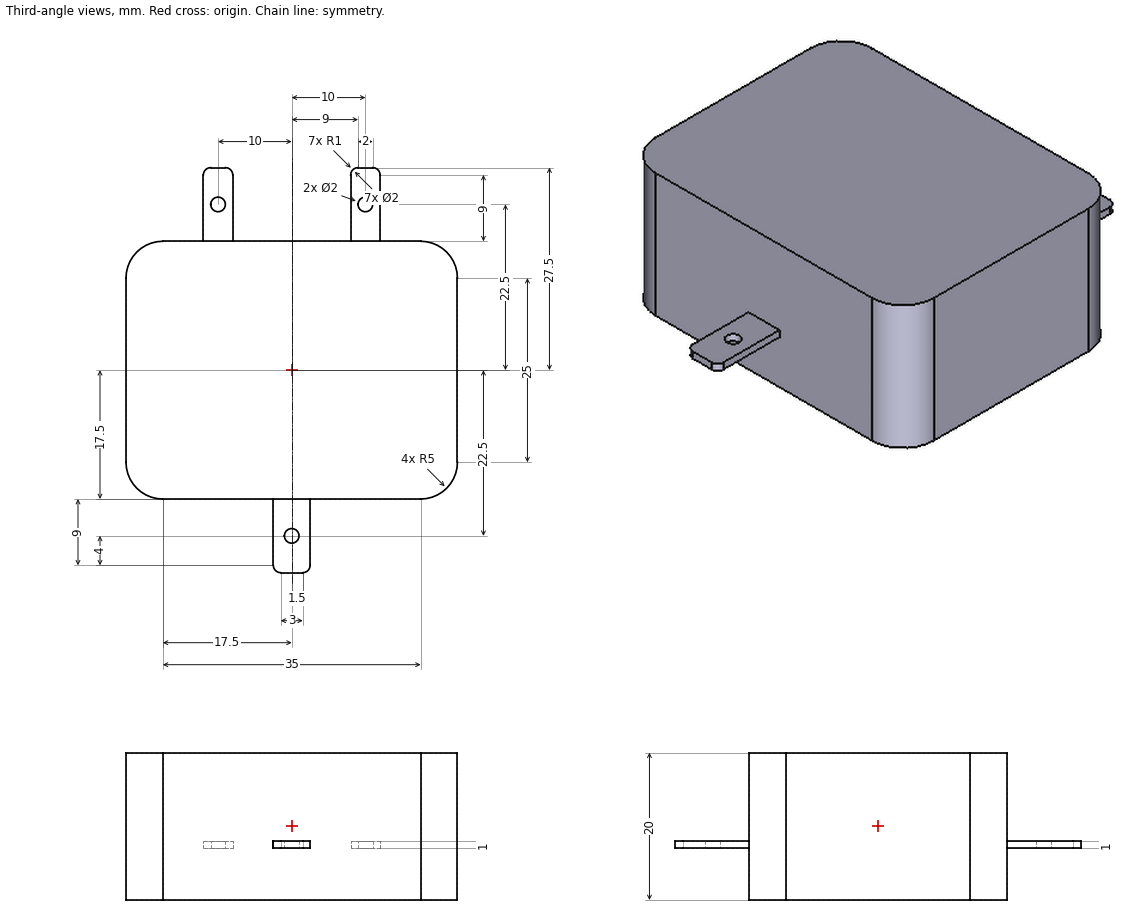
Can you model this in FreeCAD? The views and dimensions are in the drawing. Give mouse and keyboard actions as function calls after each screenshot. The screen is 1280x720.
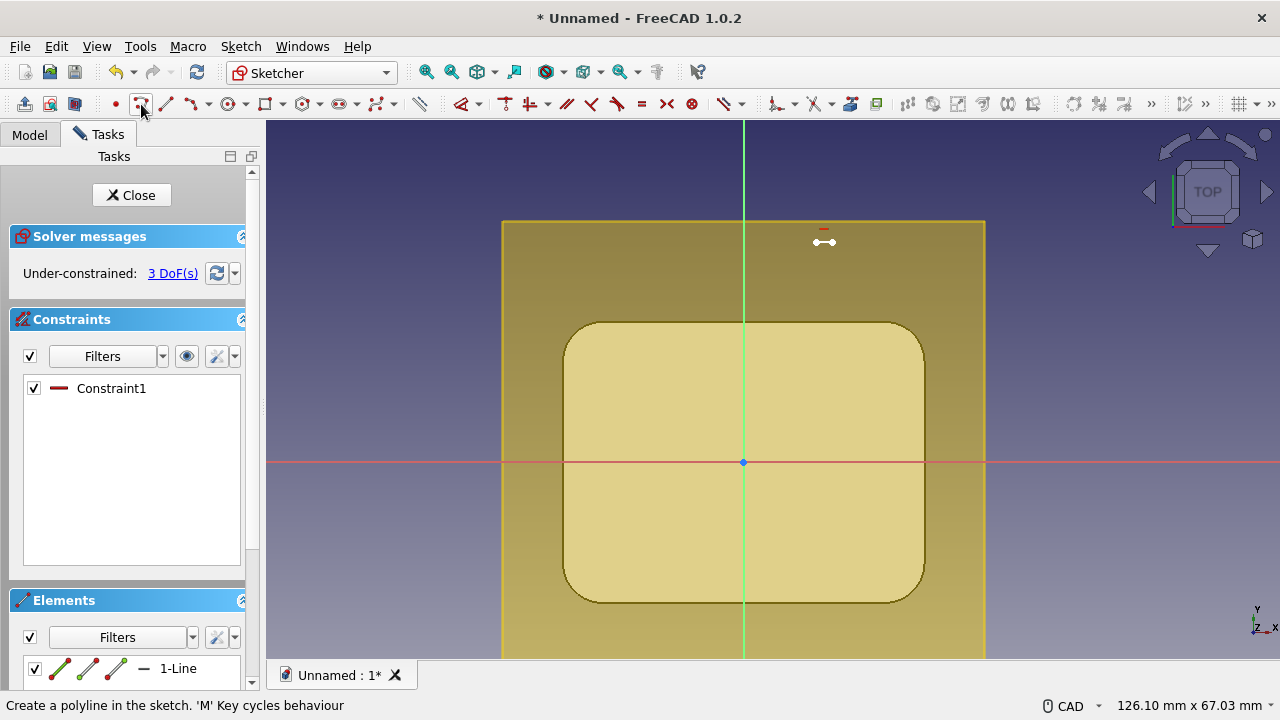
scroll(840, 249, up, 2)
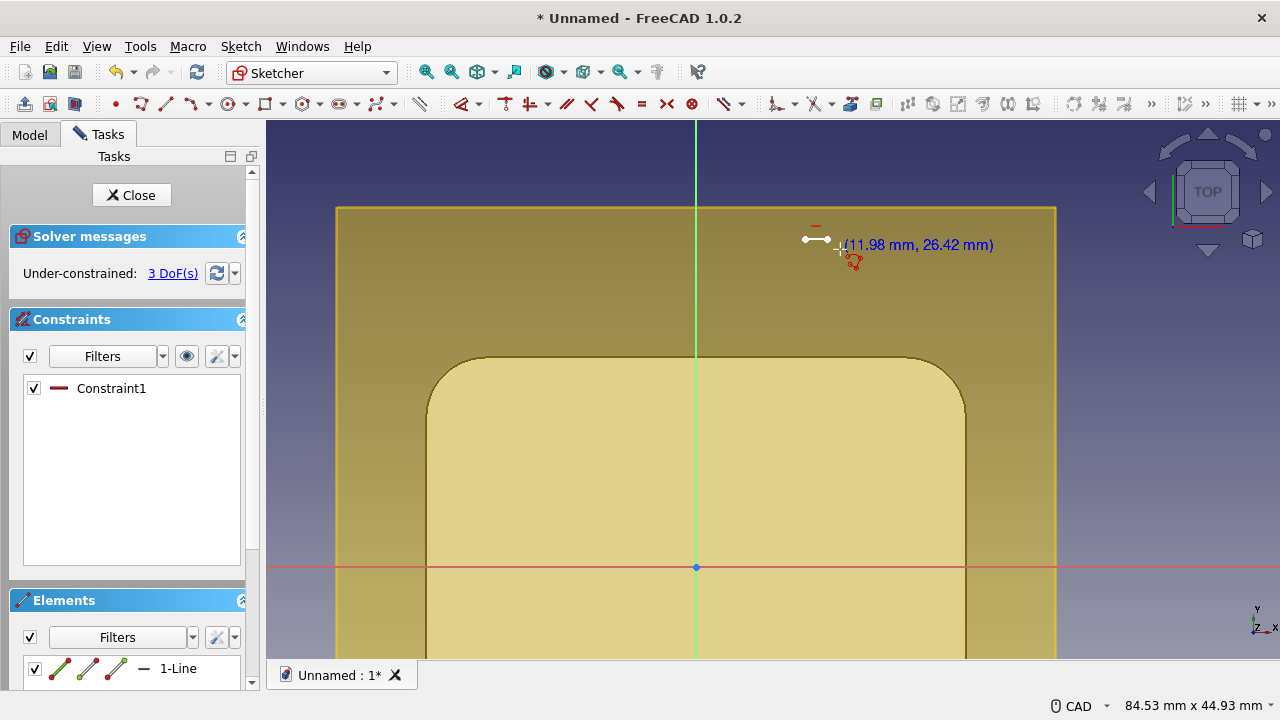
click(840, 249)
click(840, 357)
click(792, 357)
click(792, 249)
right_click(792, 249)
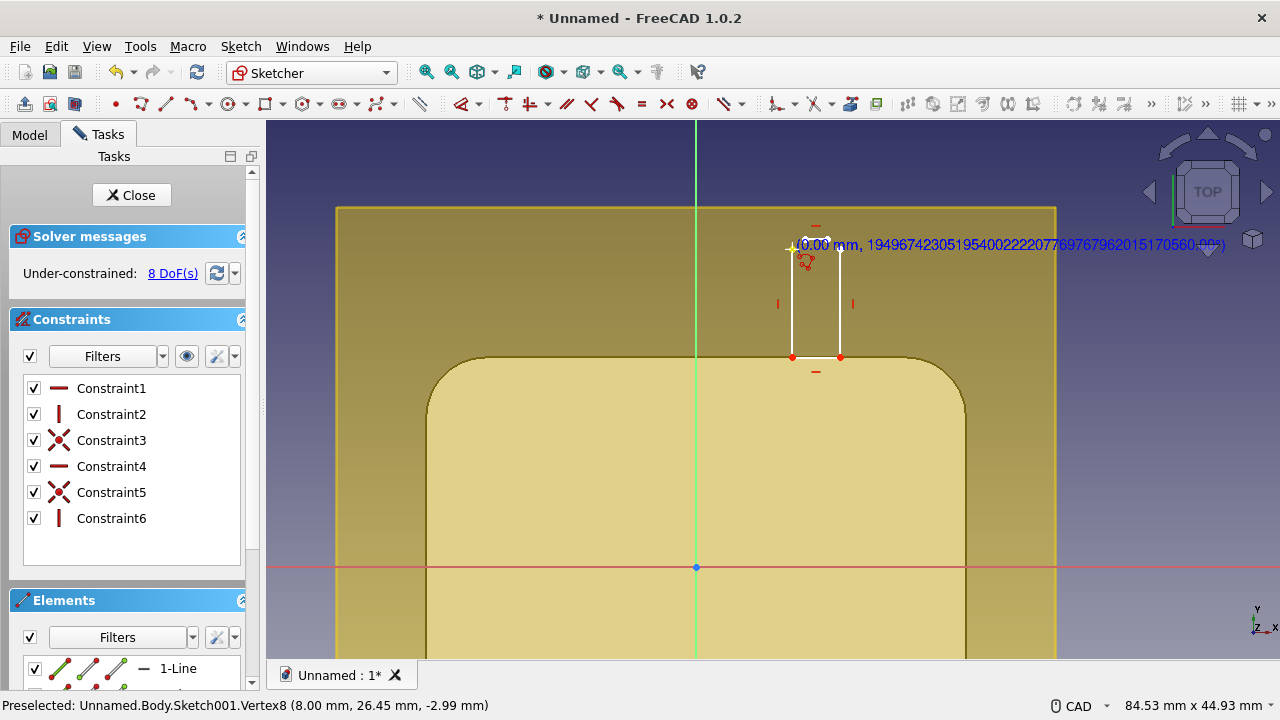
click(190, 104)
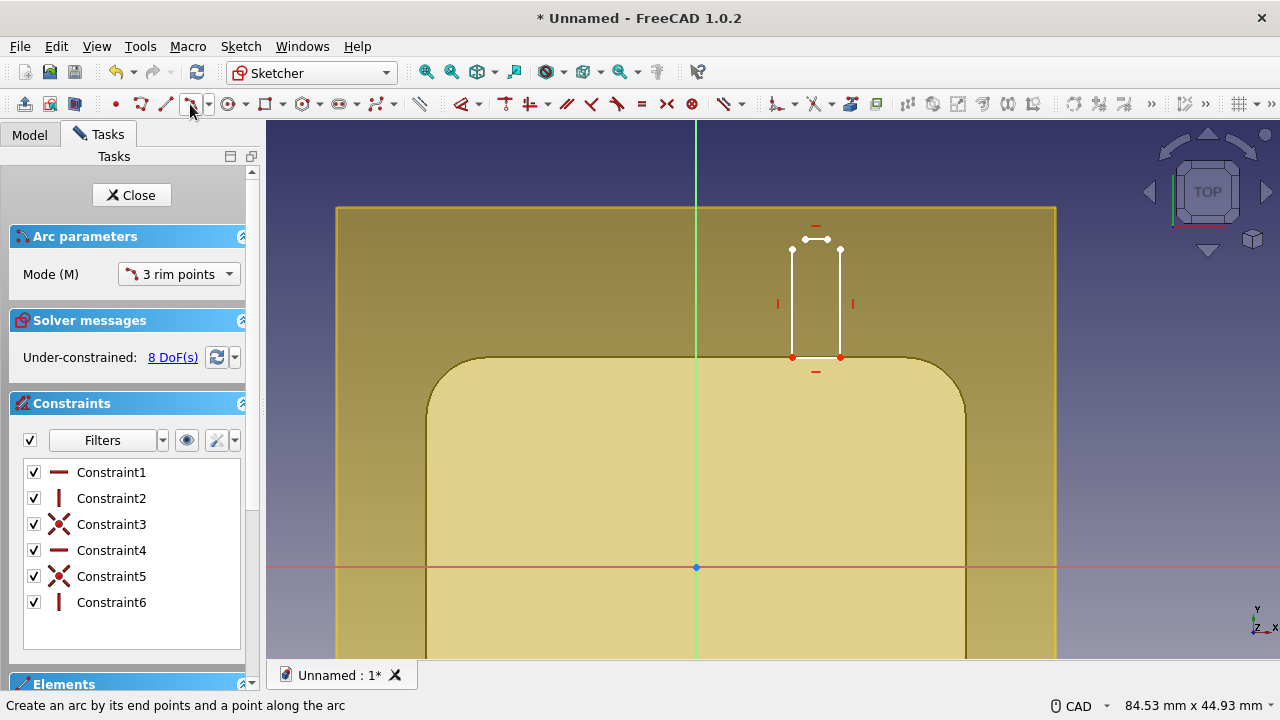
scroll(828, 237, up, 2)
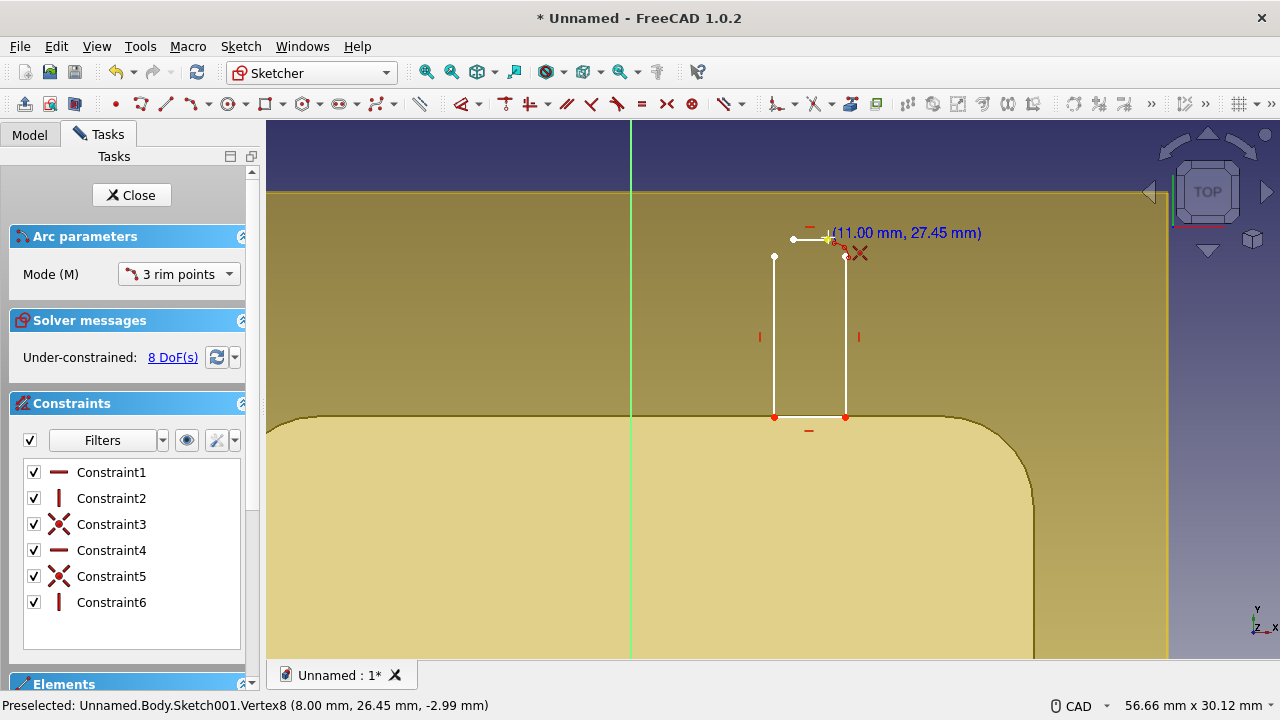
click(827, 240)
click(846, 256)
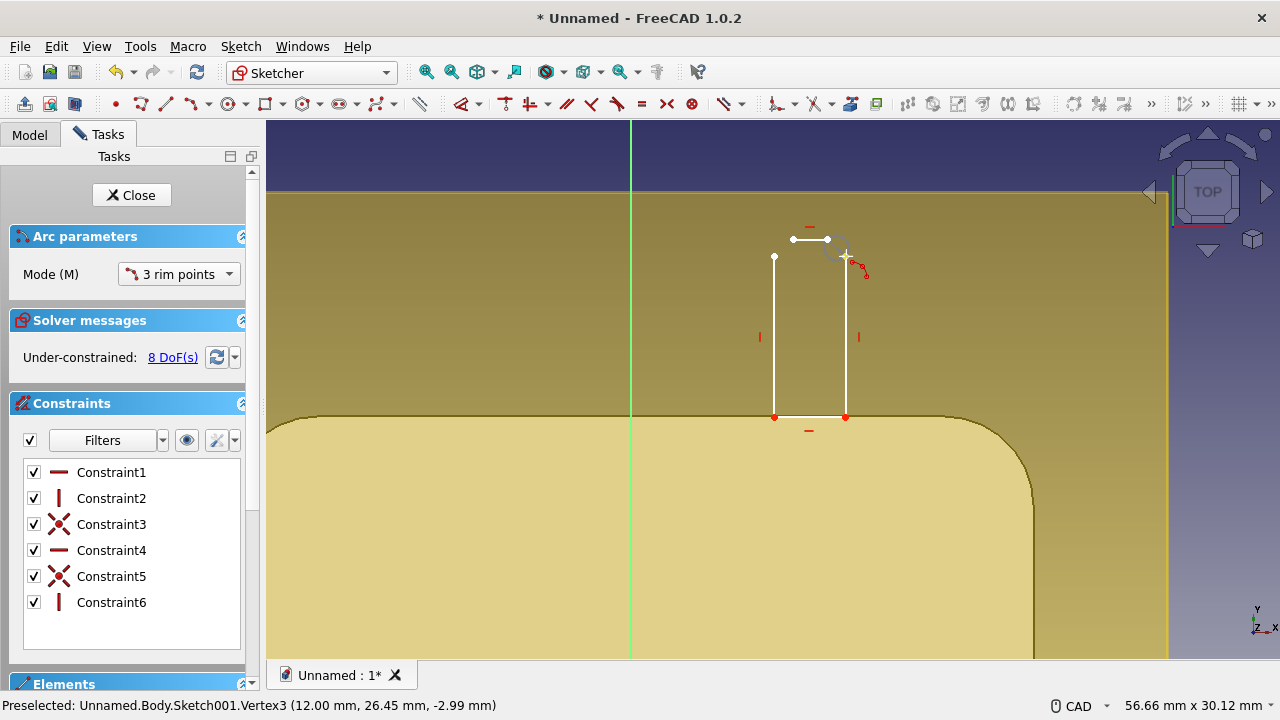
scroll(840, 243, up, 6)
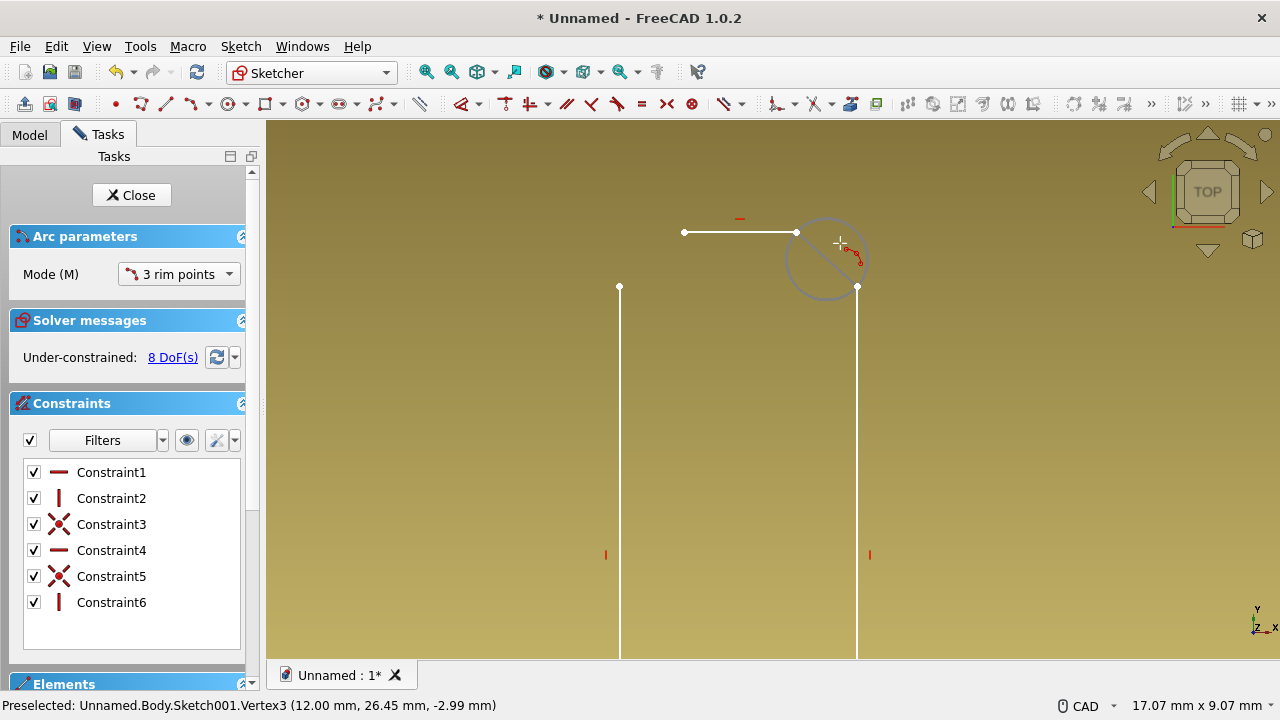
click(840, 242)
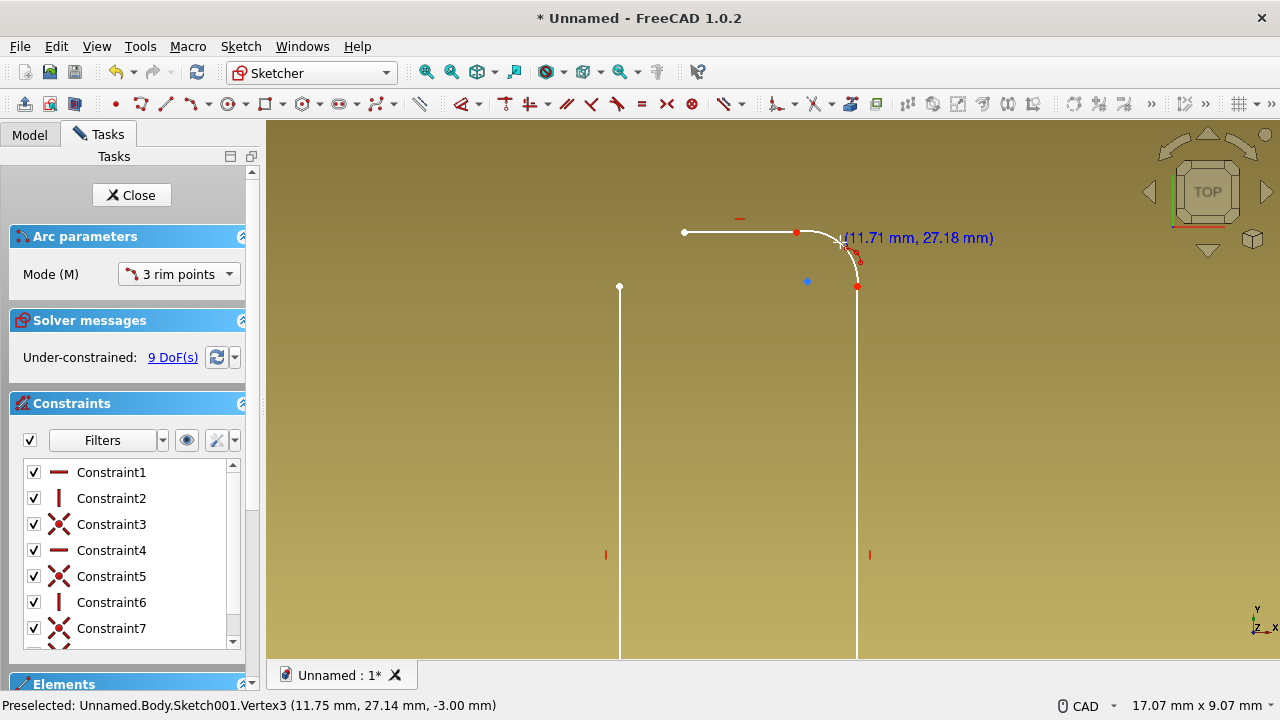
scroll(774, 207, down, 11)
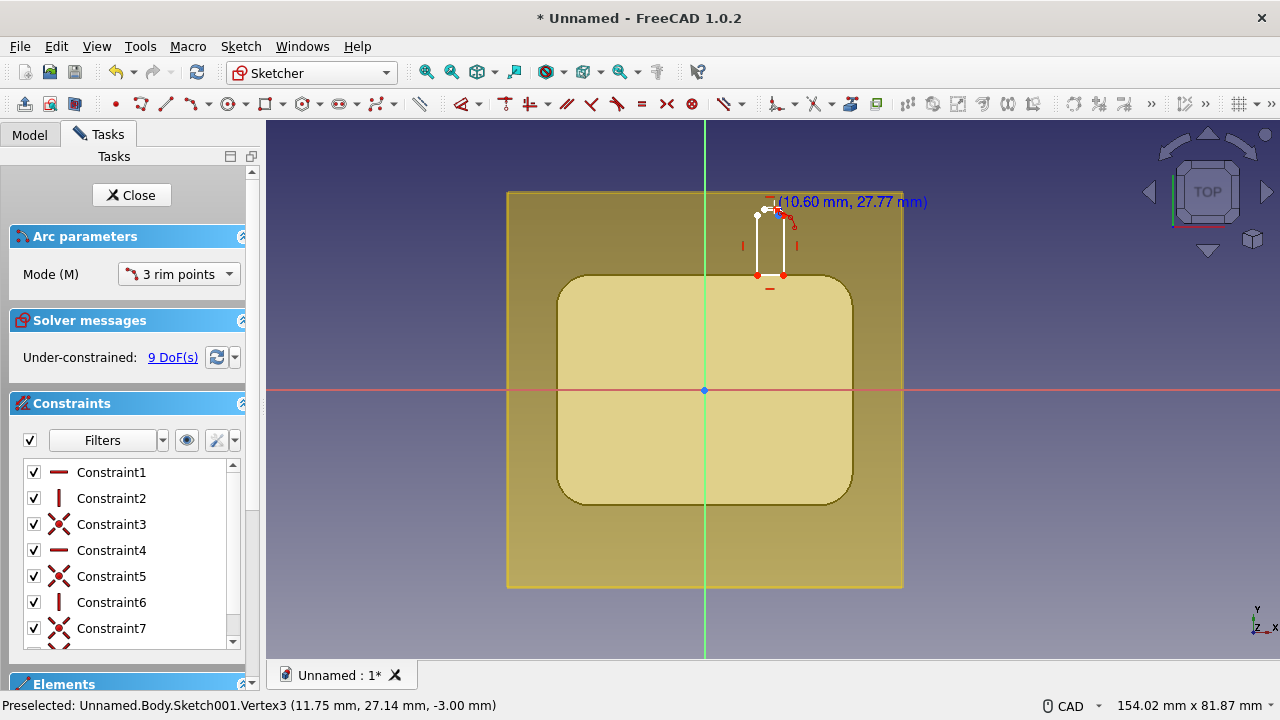
scroll(757, 216, up, 3)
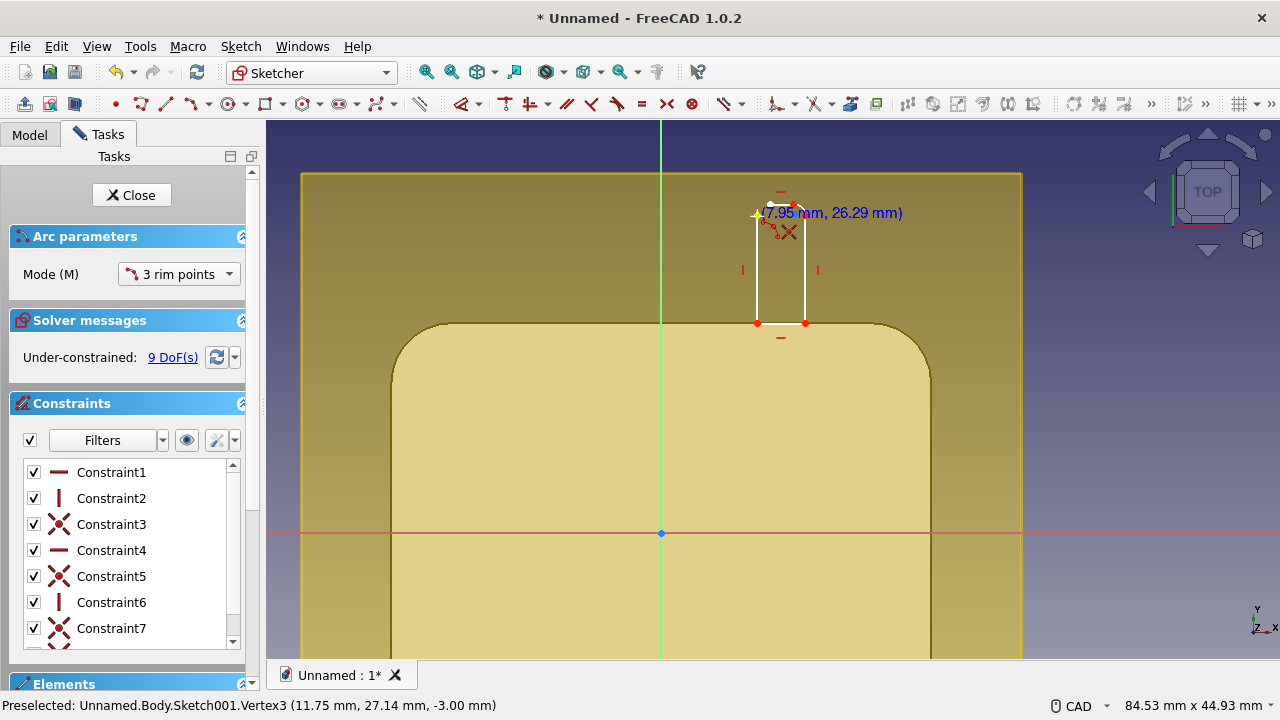
click(757, 216)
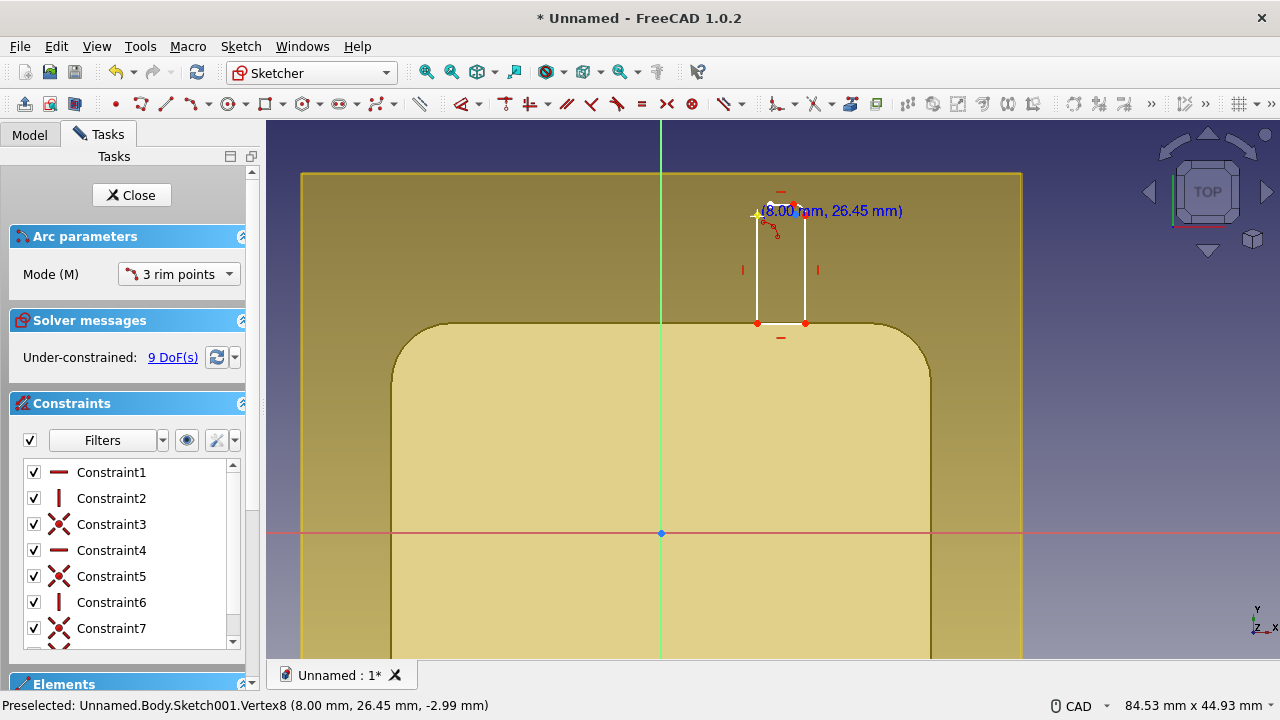
scroll(769, 203, up, 2)